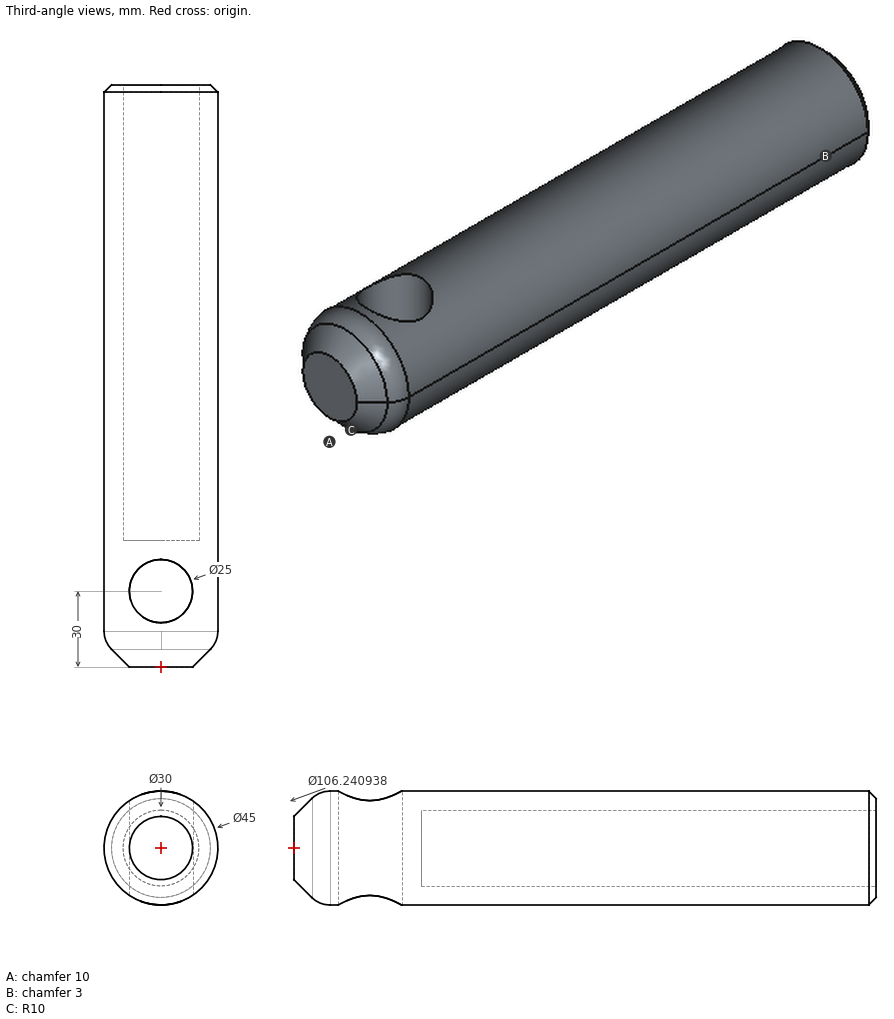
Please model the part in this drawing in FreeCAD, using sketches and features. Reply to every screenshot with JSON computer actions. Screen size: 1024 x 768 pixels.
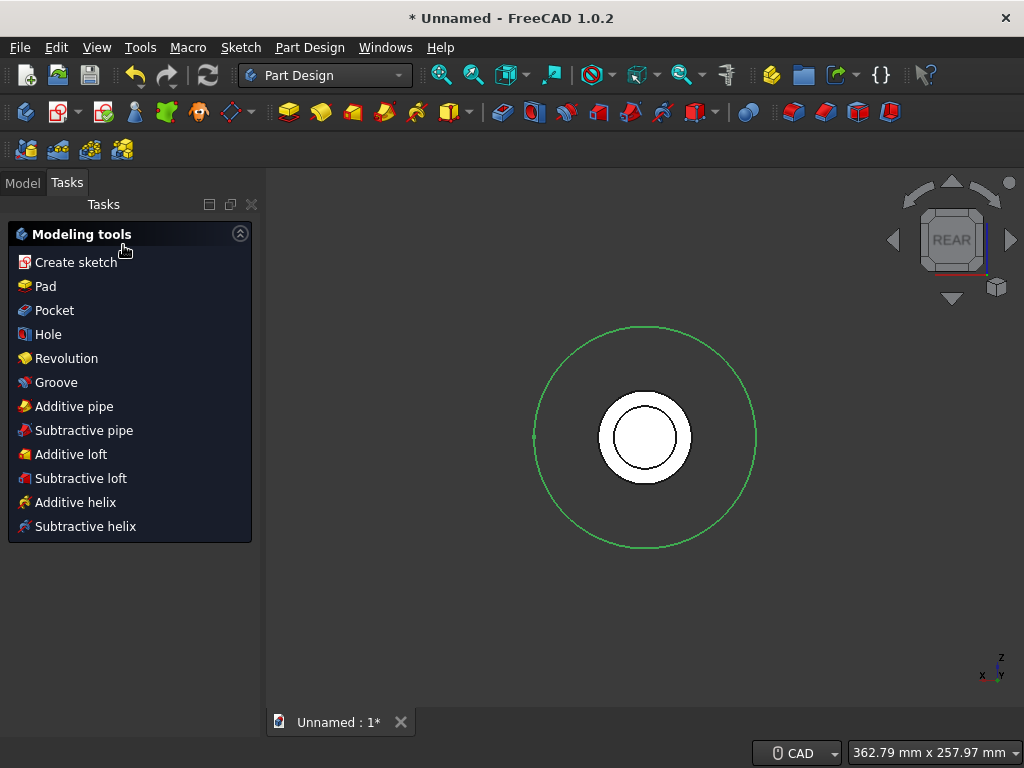
{"action": "left_click", "coordinate": [504, 112]}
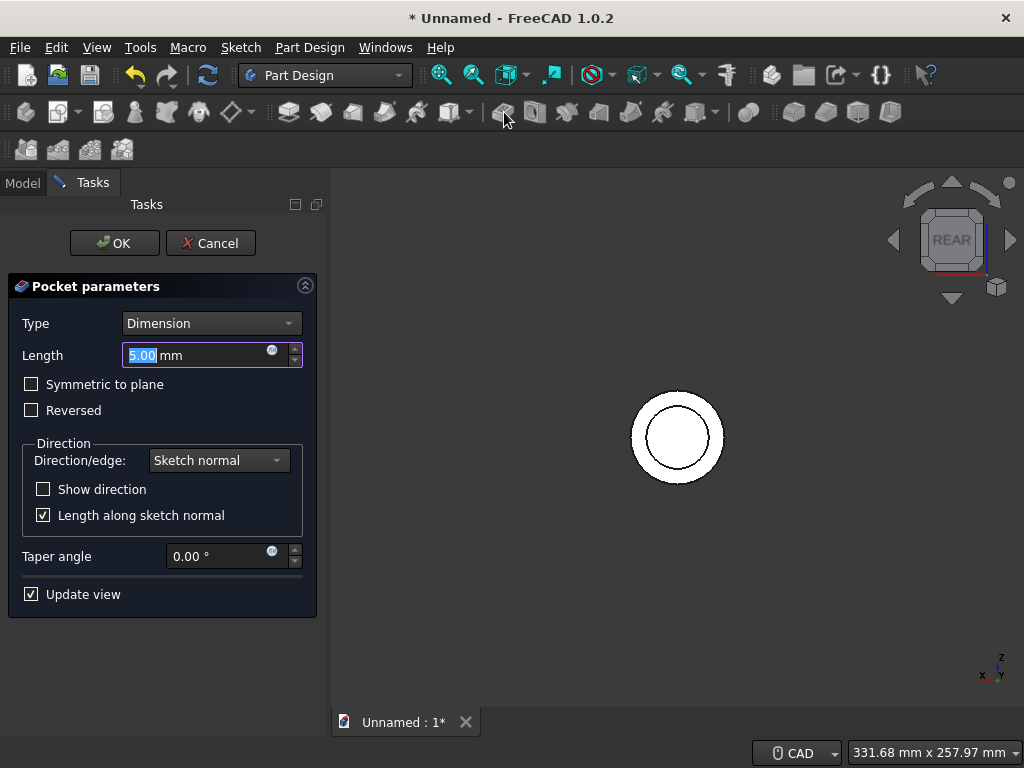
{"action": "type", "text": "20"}
{"action": "key", "text": "Tab"}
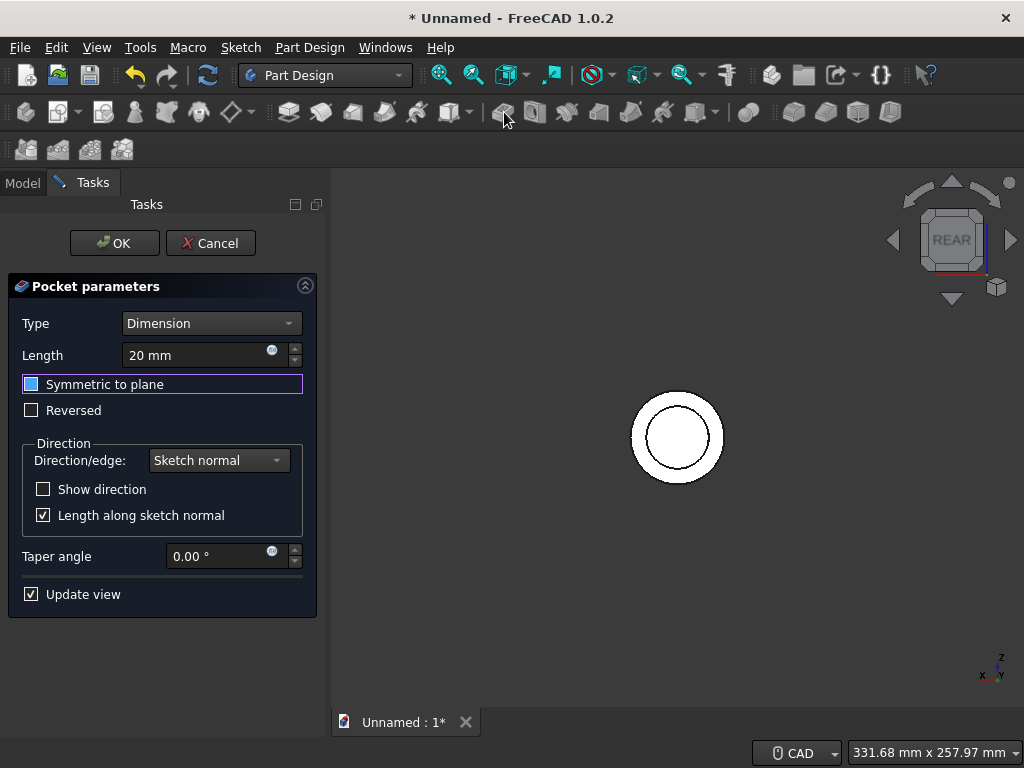
{"action": "left_click", "coordinate": [115, 243]}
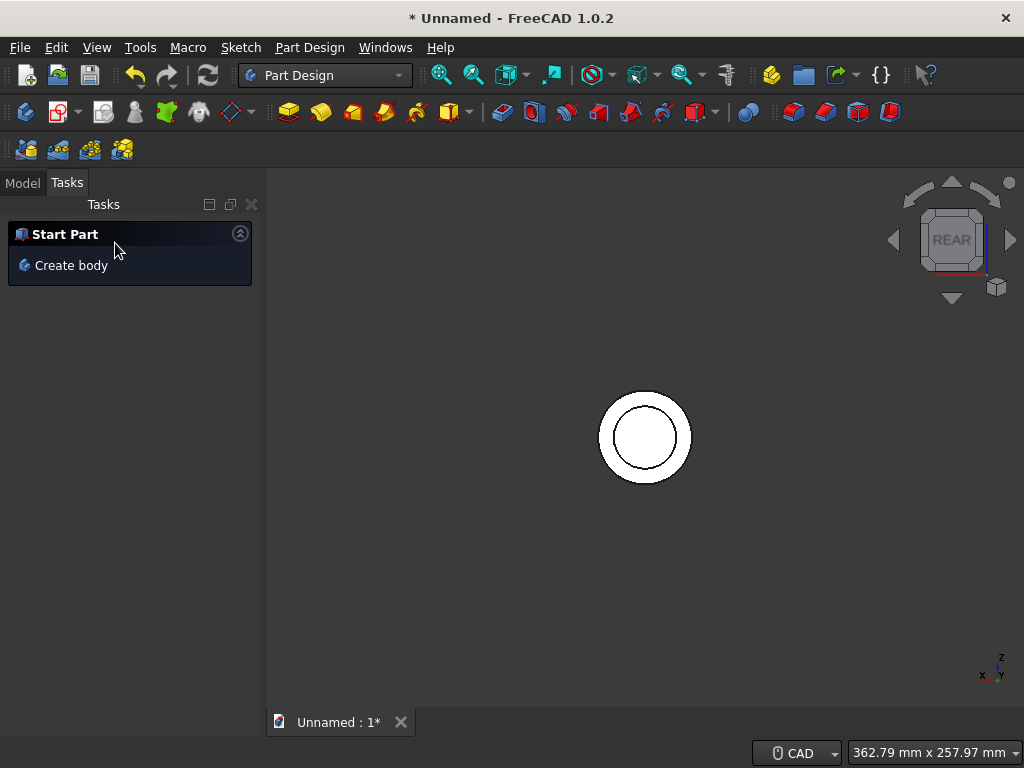
{"action": "key", "text": "v f"}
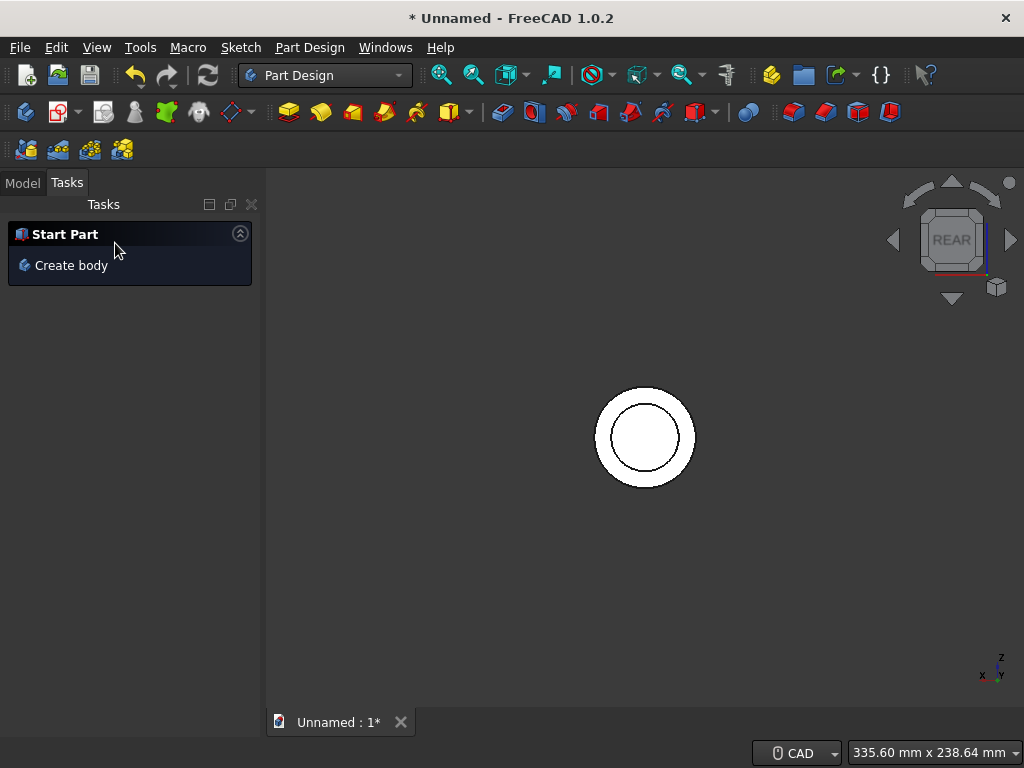
{"action": "key", "text": "0"}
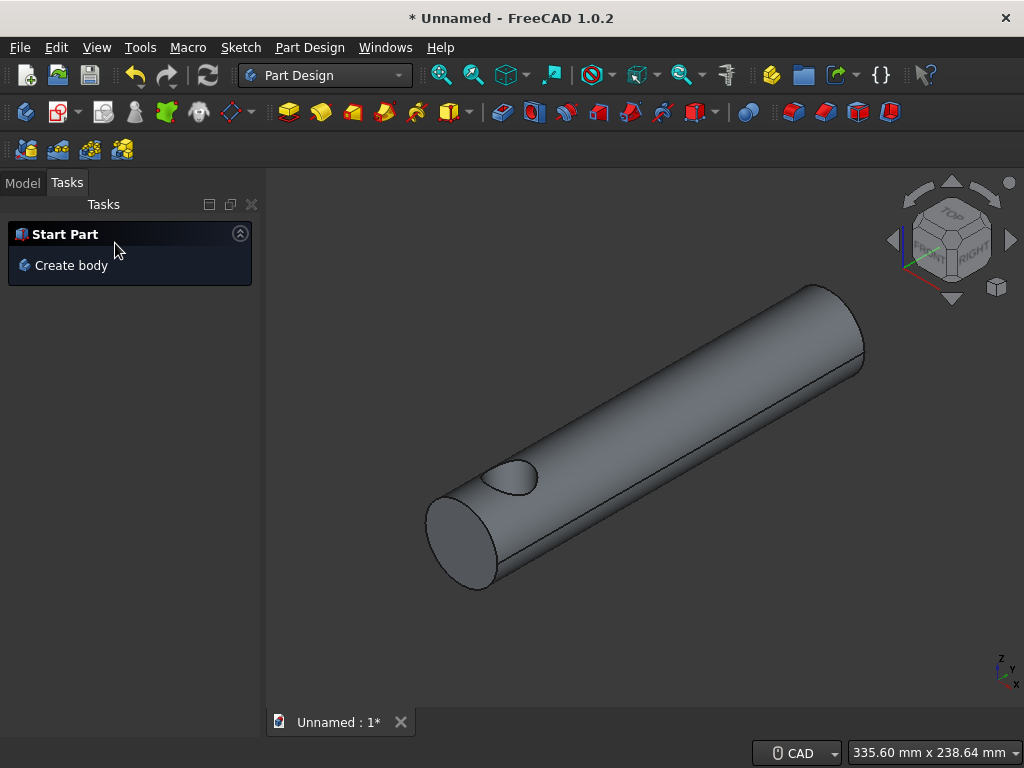
{"action": "left_click", "coordinate": [450, 497]}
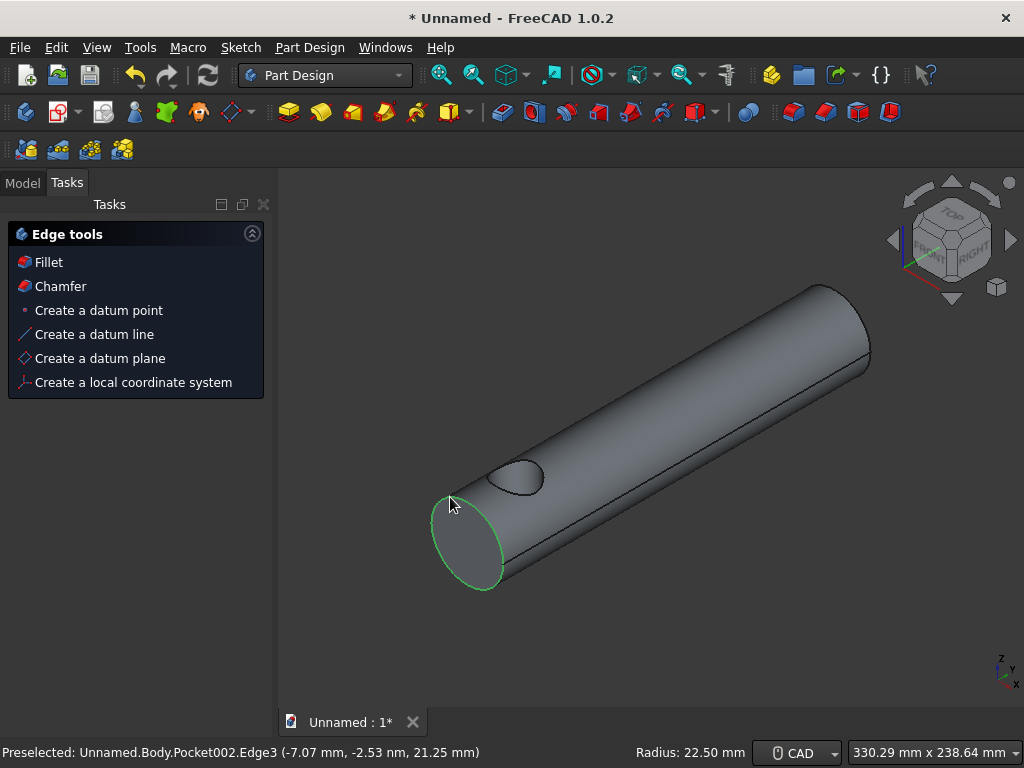
{"action": "left_click", "coordinate": [826, 112]}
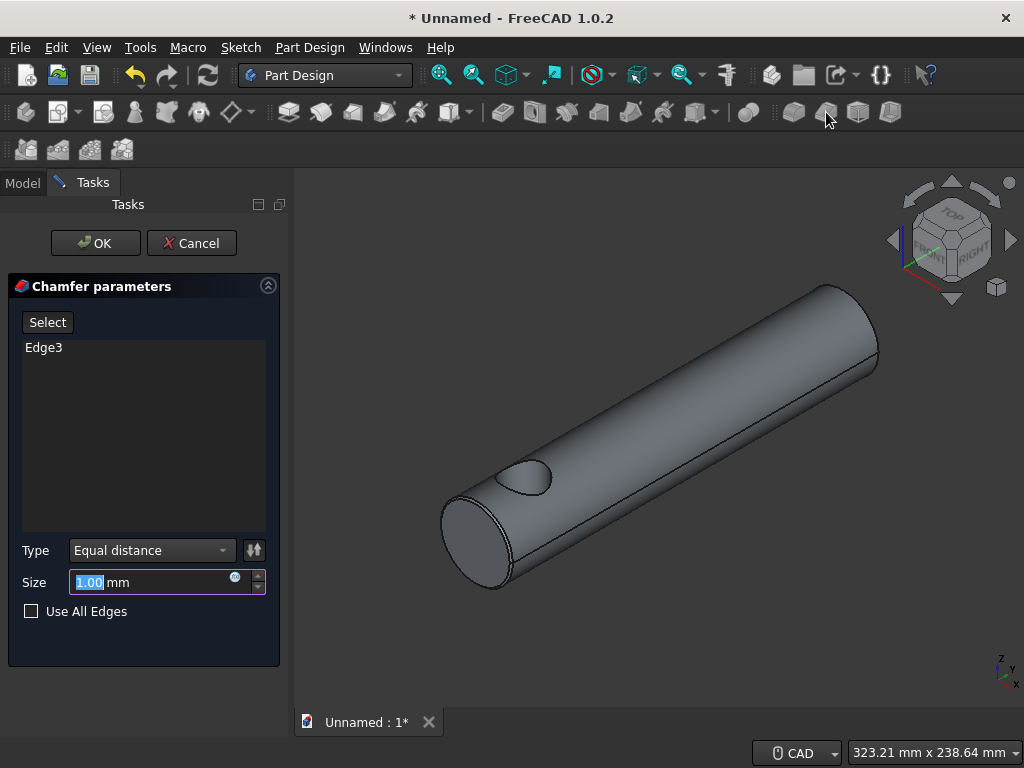
{"action": "type", "text": "10"}
{"action": "key", "text": "Tab"}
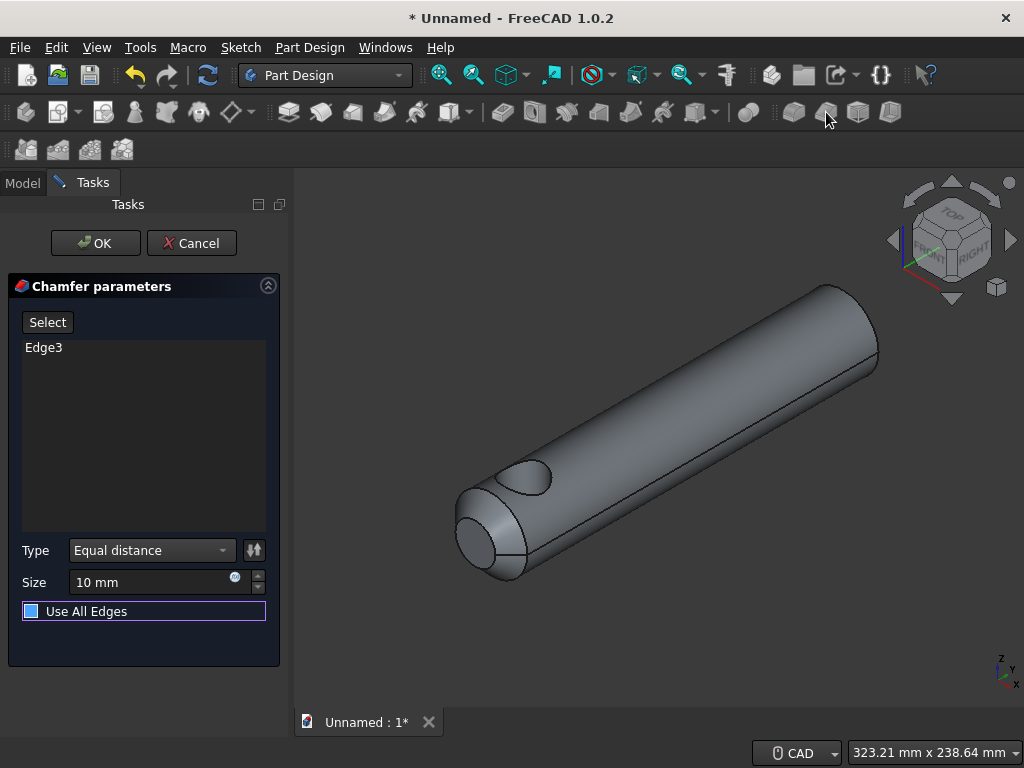
{"action": "left_click", "coordinate": [96, 243]}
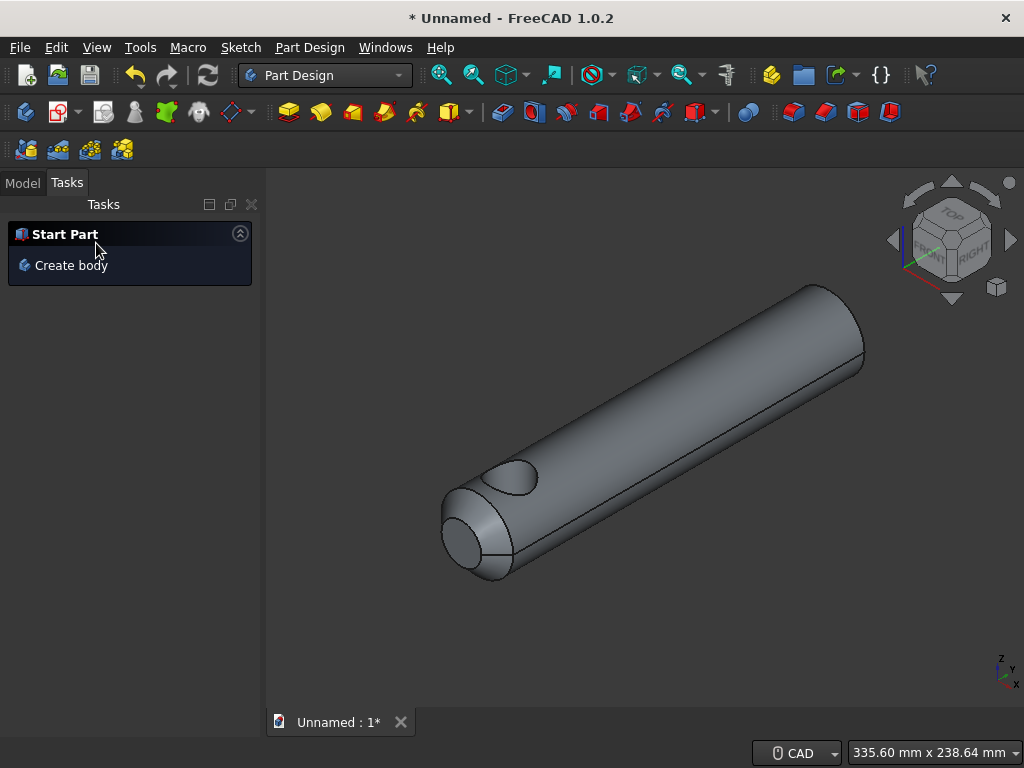
{"action": "key", "text": "2"}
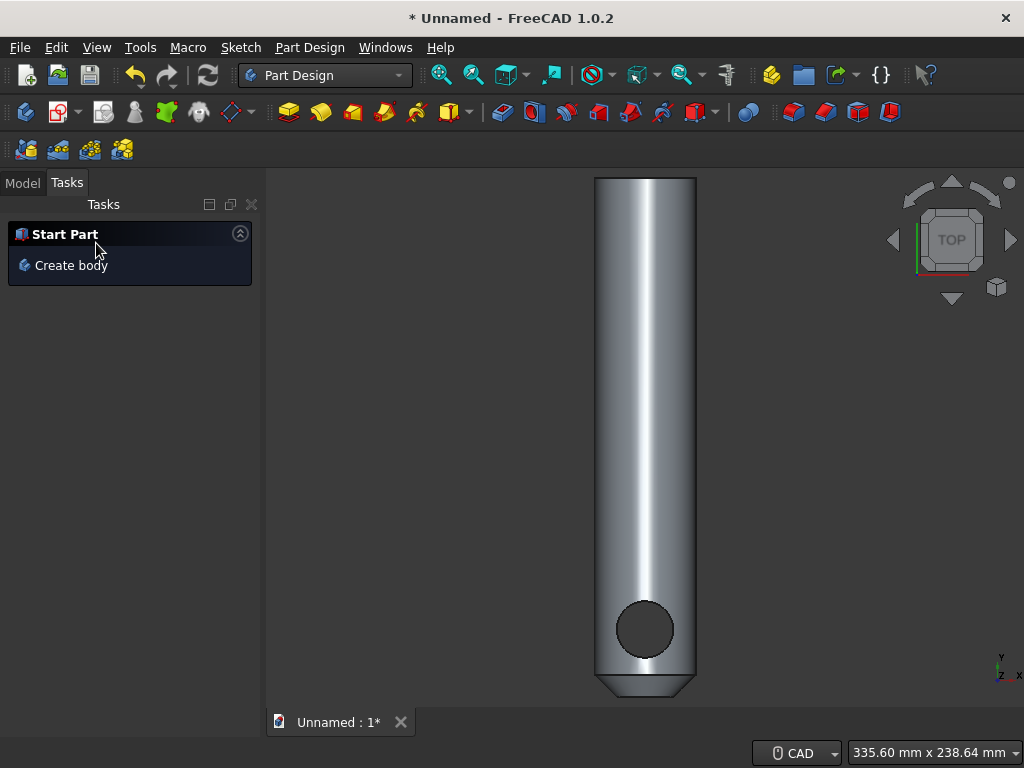
{"action": "key", "text": "0"}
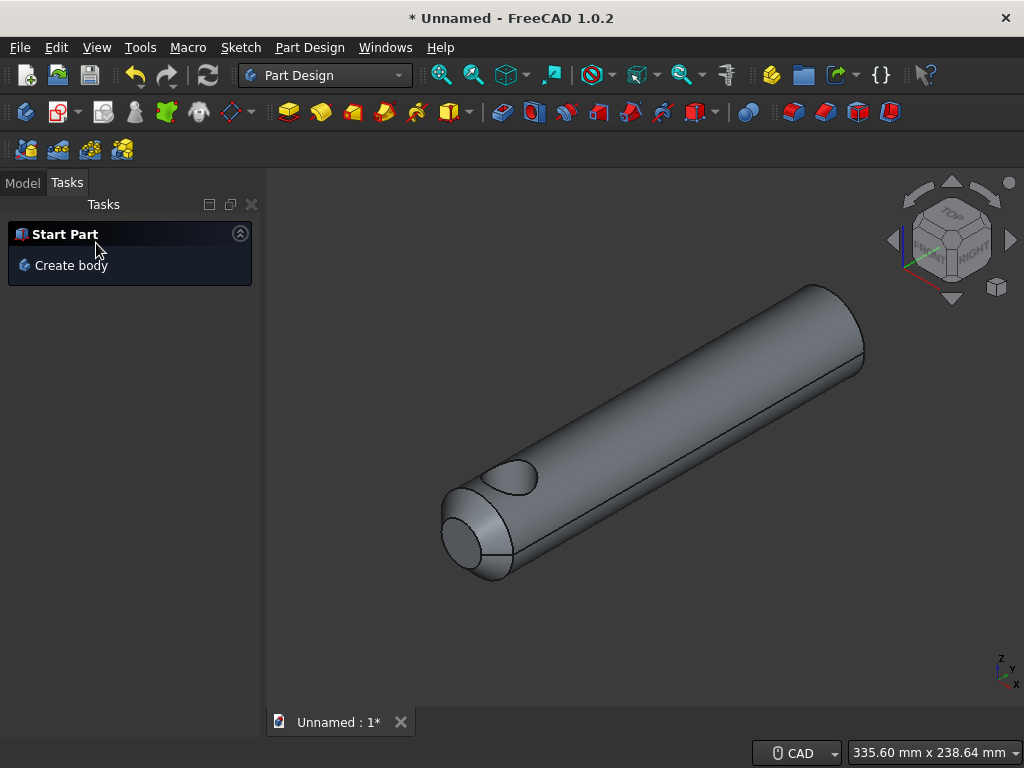
{"action": "key", "text": "1"}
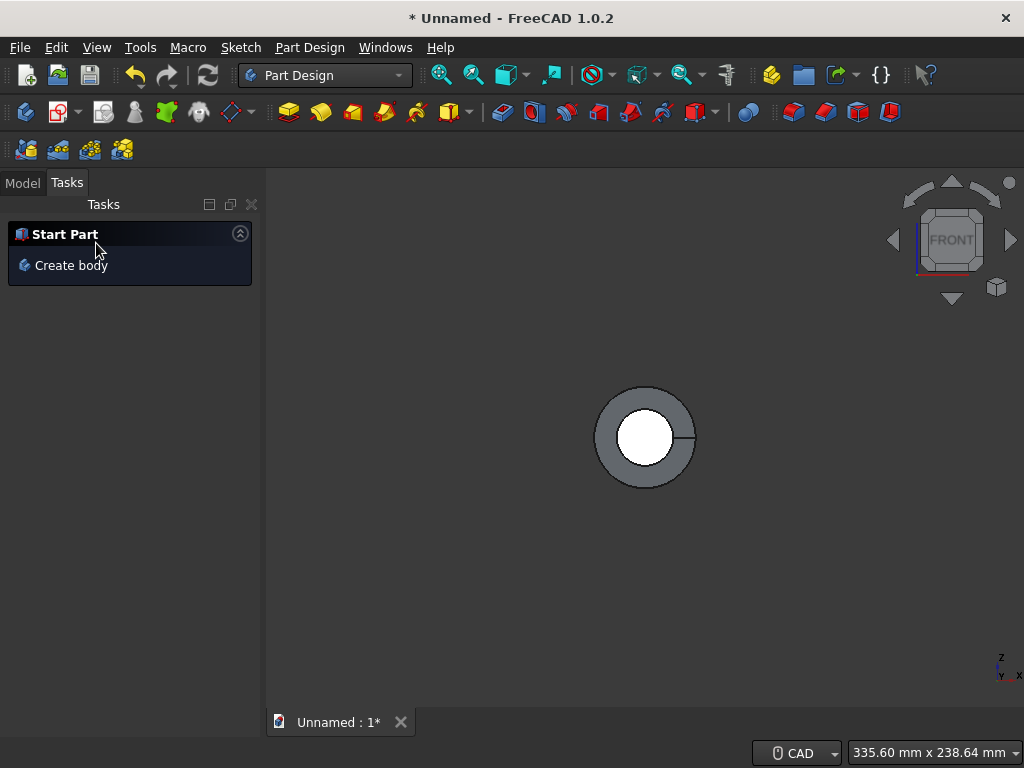
{"action": "left_click", "coordinate": [442, 76]}